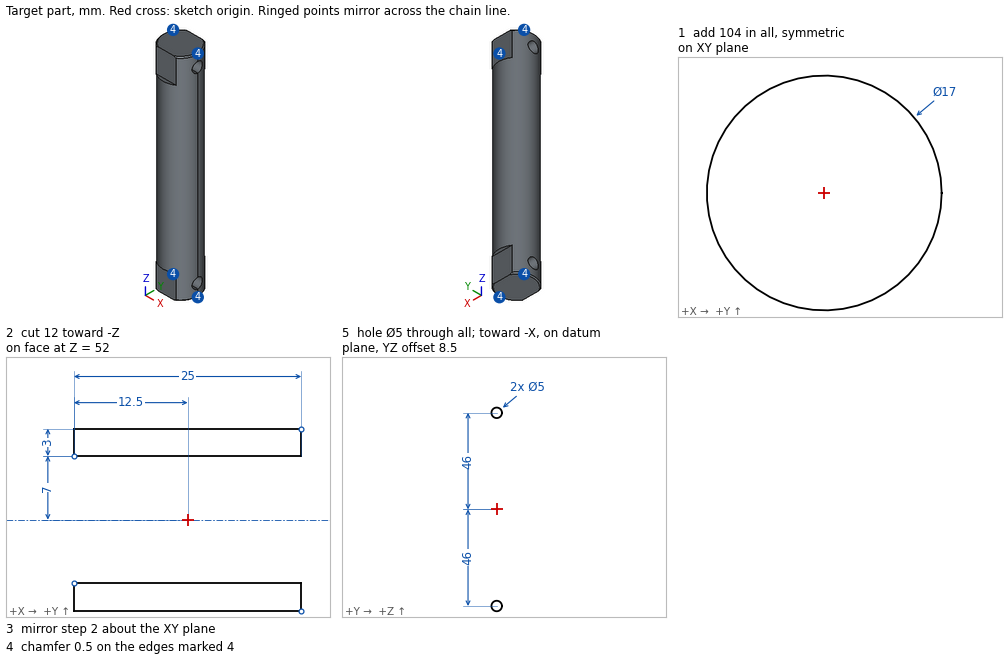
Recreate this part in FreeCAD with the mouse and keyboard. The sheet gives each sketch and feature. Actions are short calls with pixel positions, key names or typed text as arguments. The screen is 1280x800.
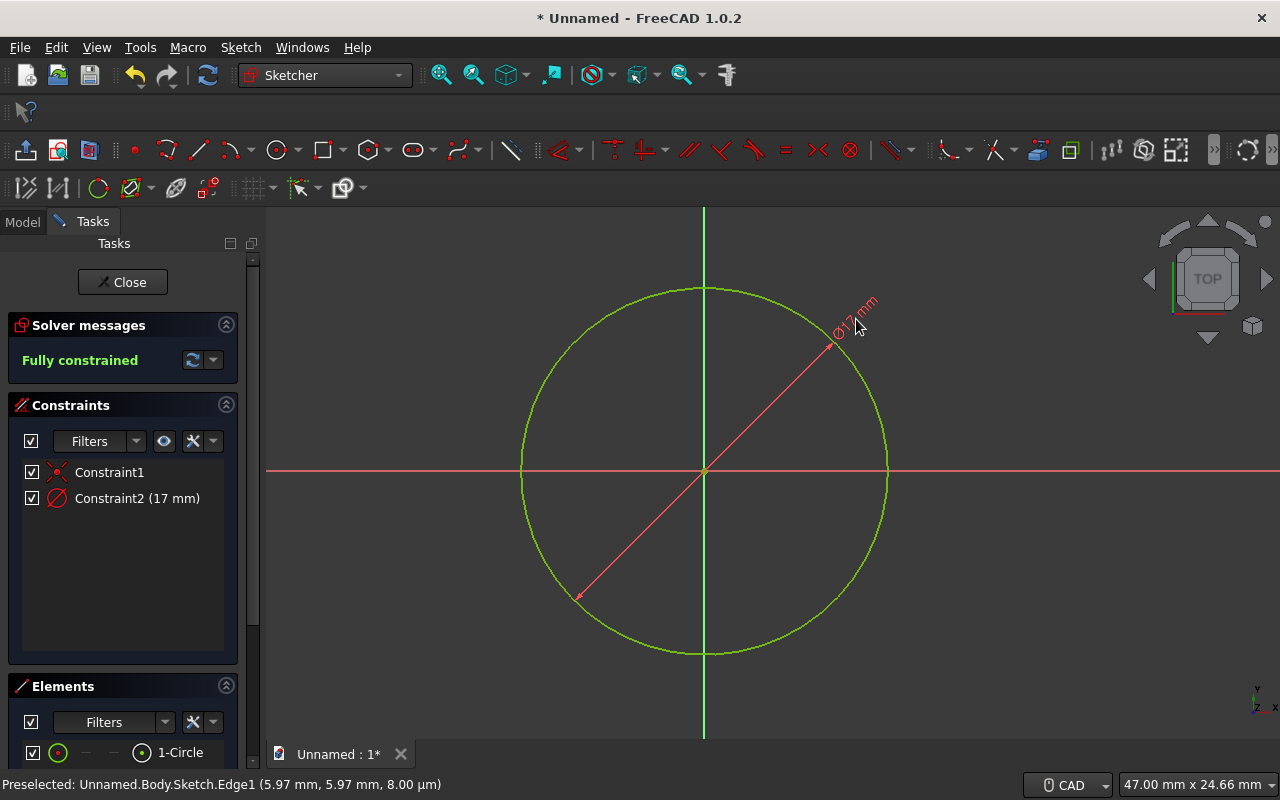
click(123, 282)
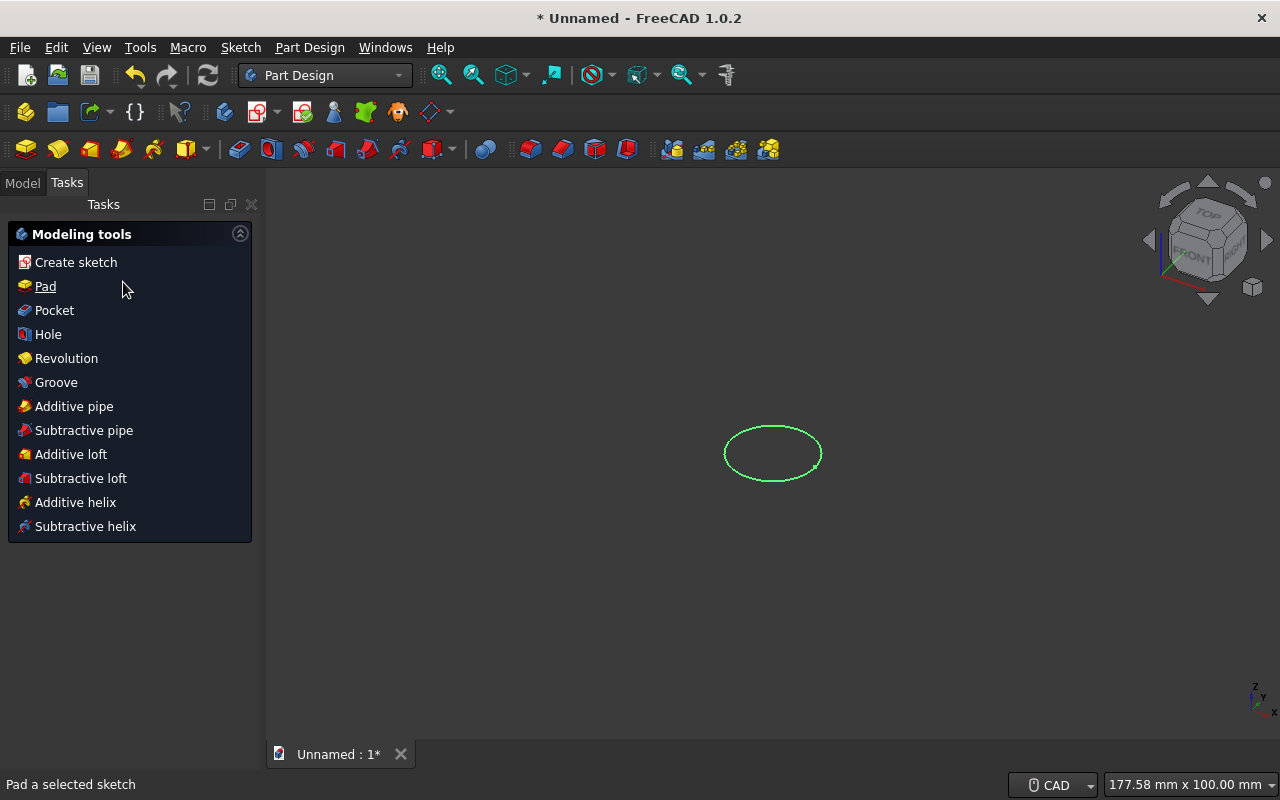
click(26, 150)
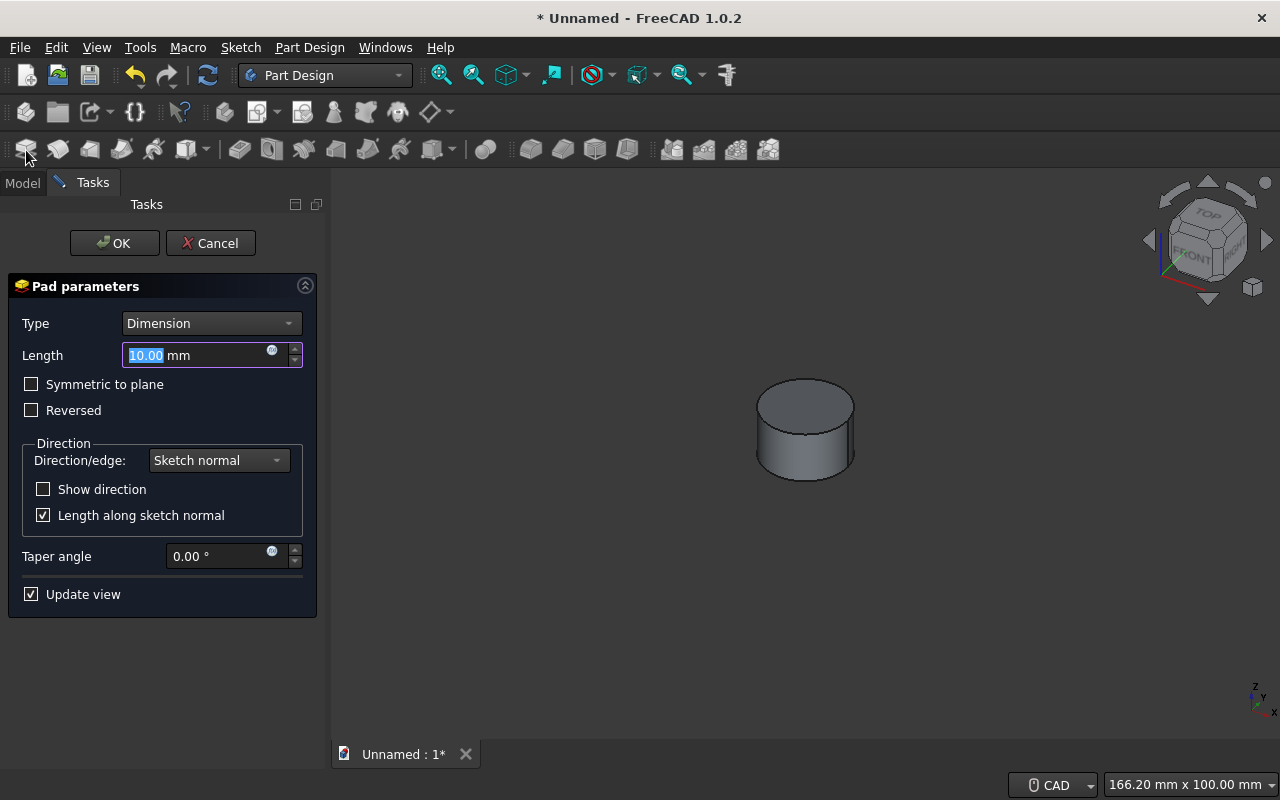
text(104)
key(Tab)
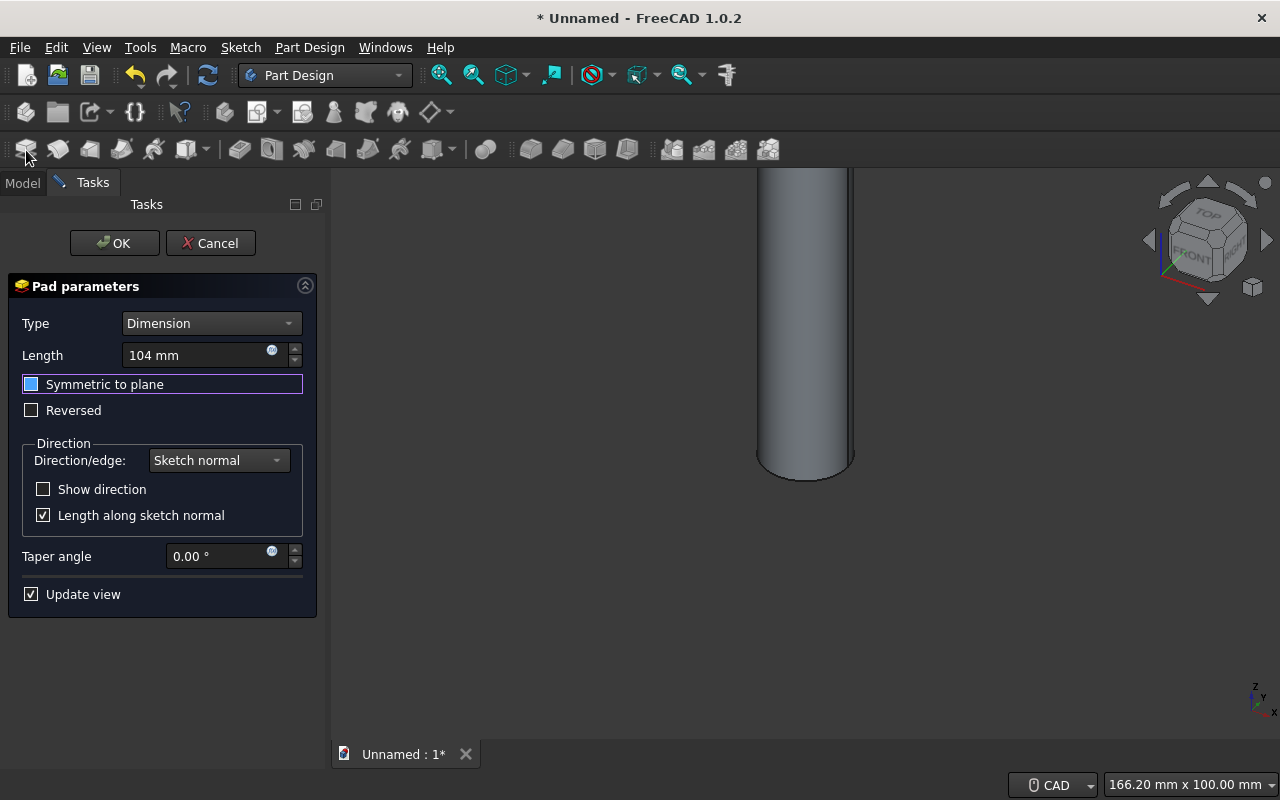
click(30, 384)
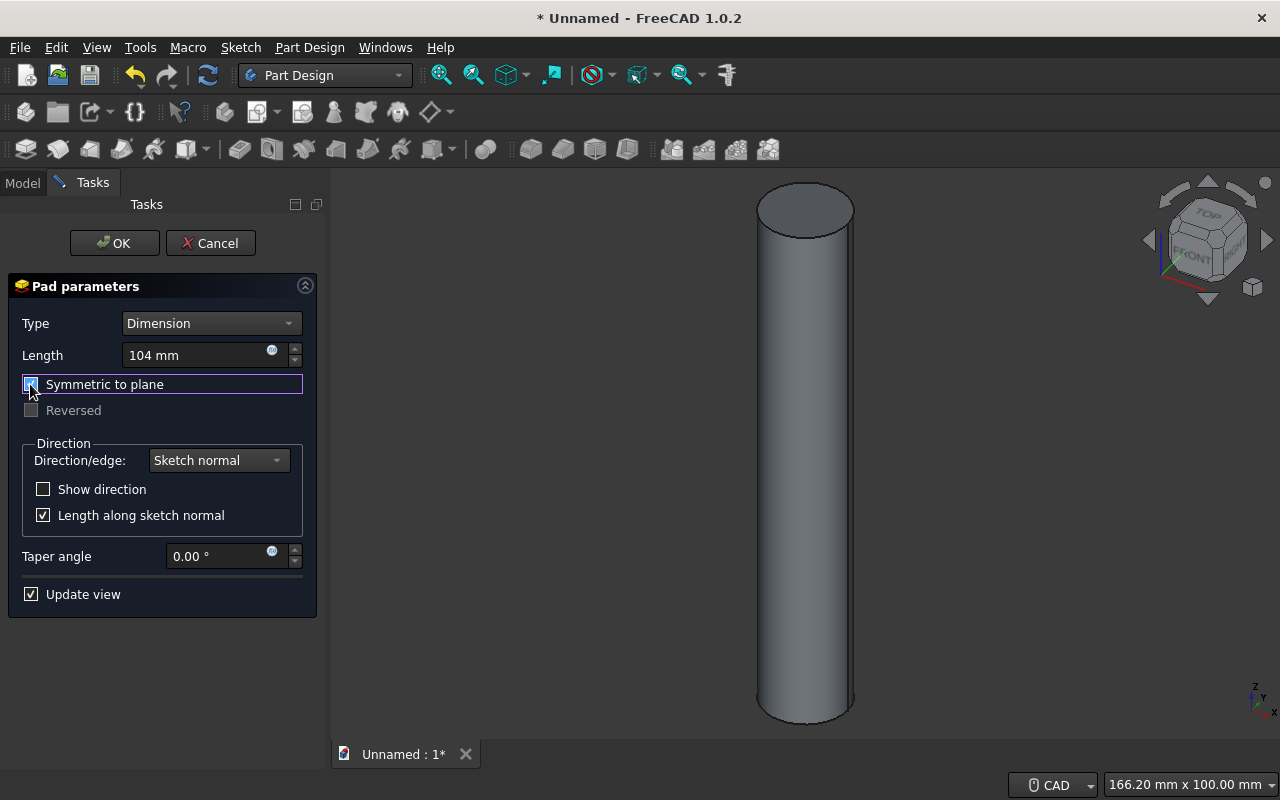
click(115, 243)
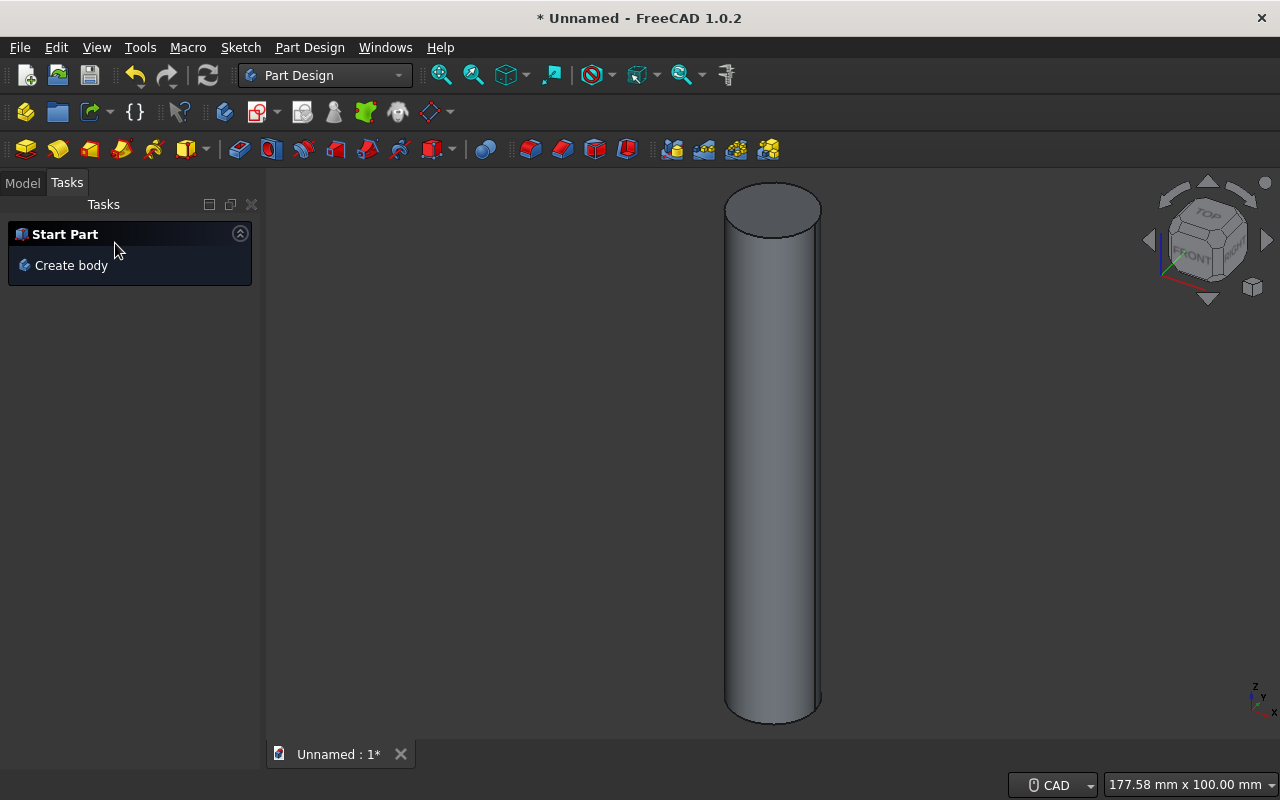
click(773, 209)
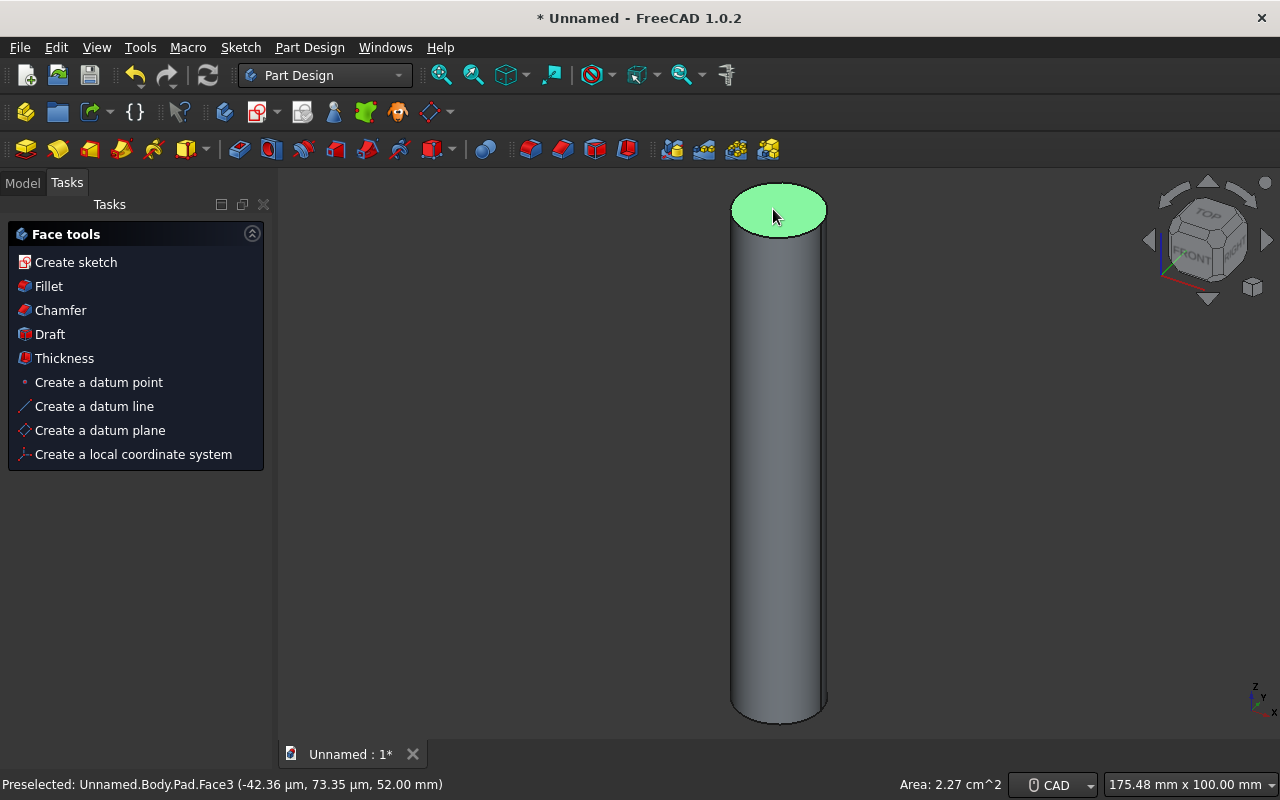
click(258, 112)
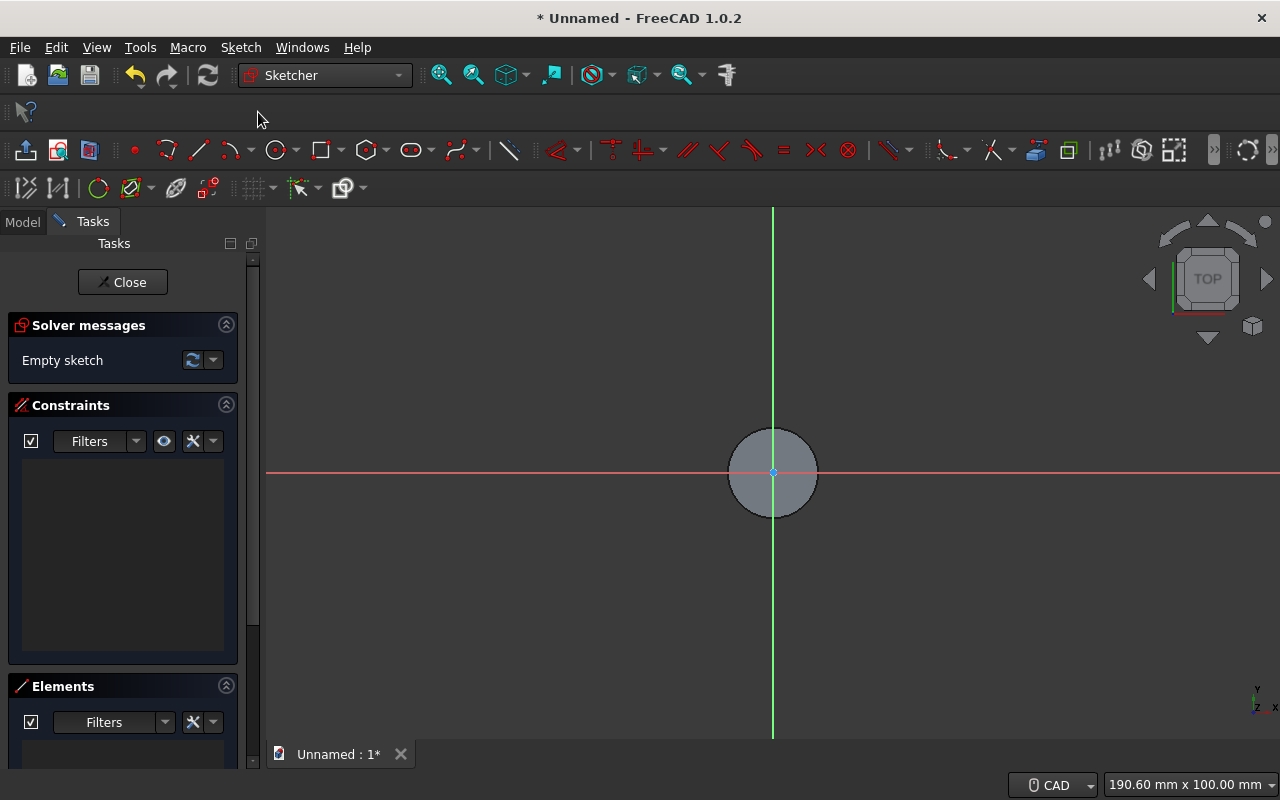
scroll(803, 473, up, 6)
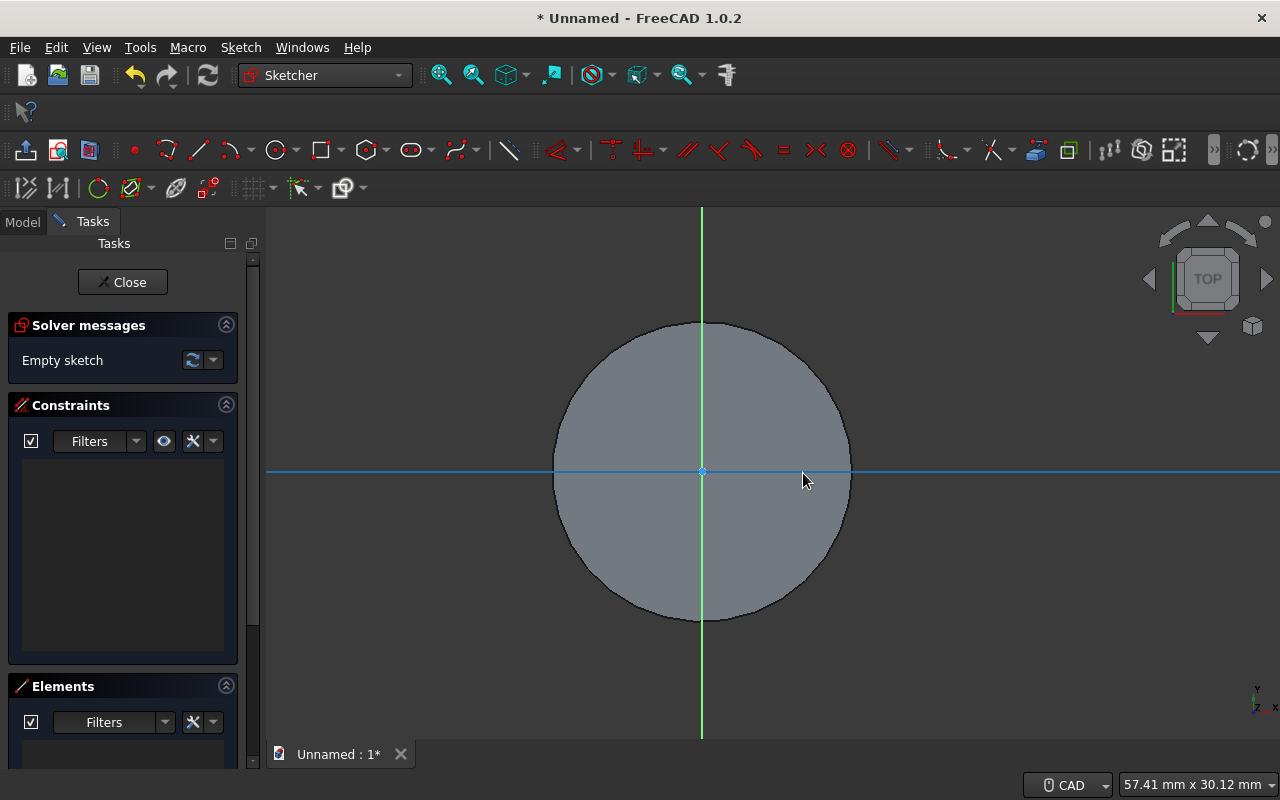
click(322, 150)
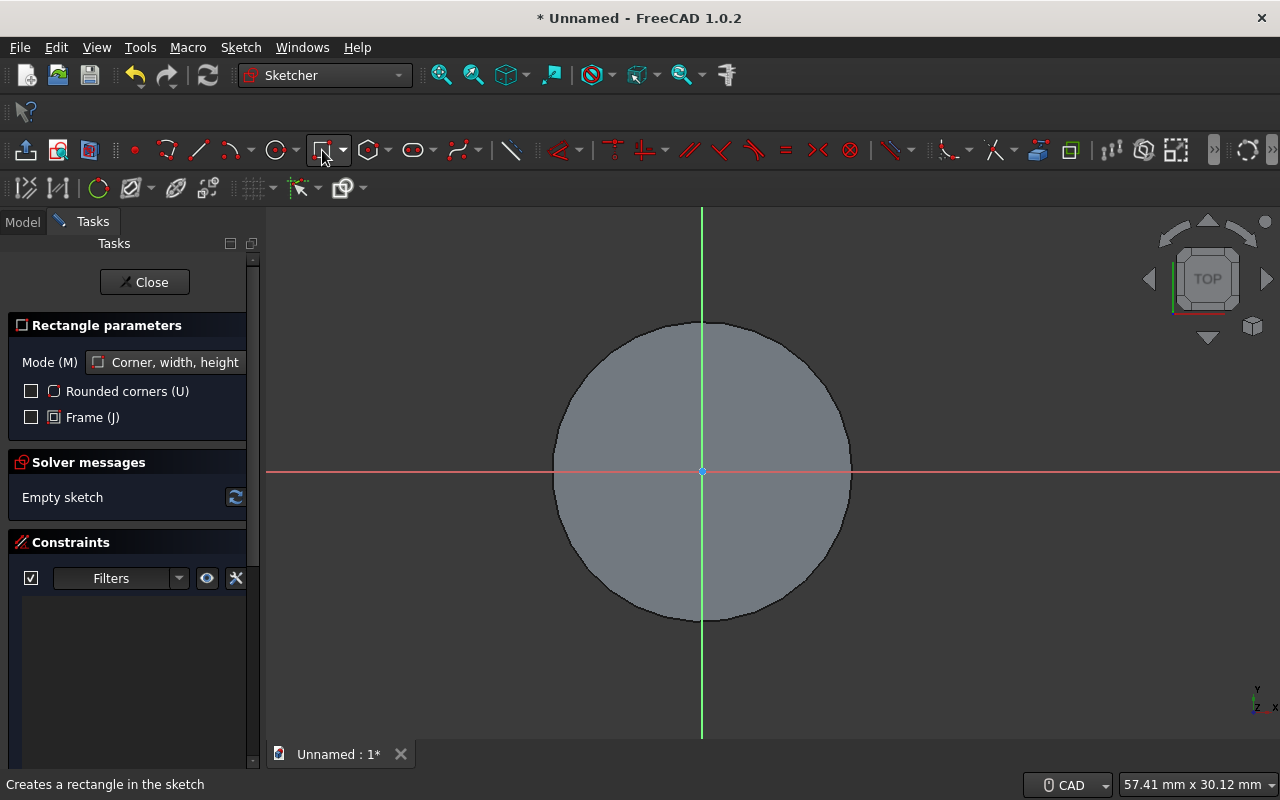
click(481, 295)
click(923, 348)